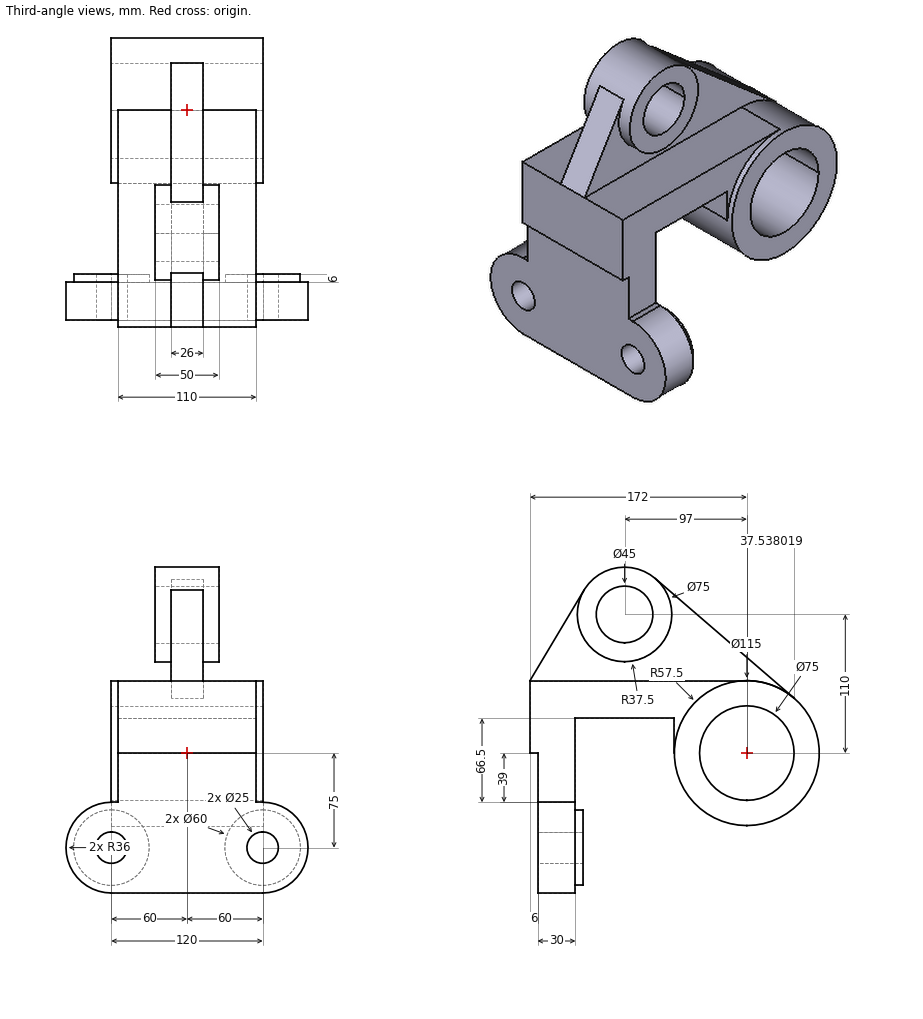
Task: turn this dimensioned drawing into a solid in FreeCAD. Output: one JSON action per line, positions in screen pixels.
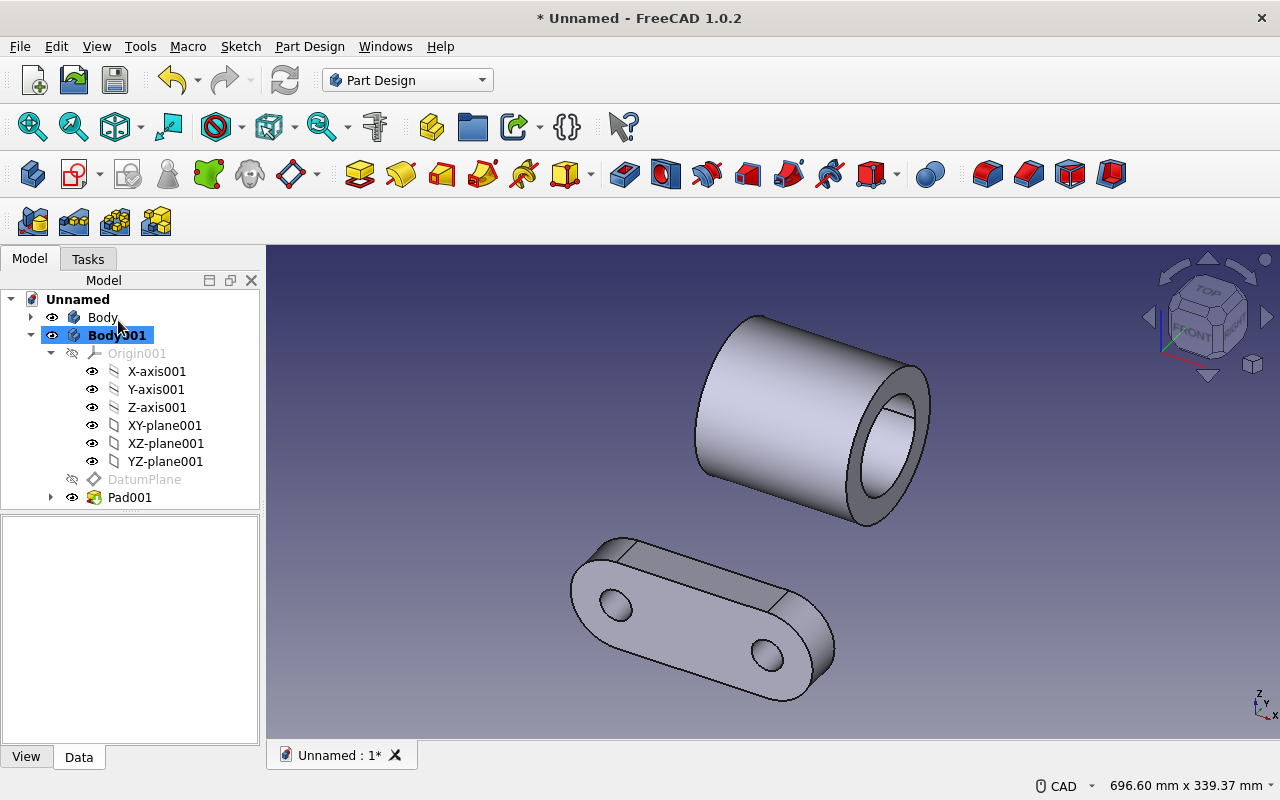
{"action": "key", "text": "4"}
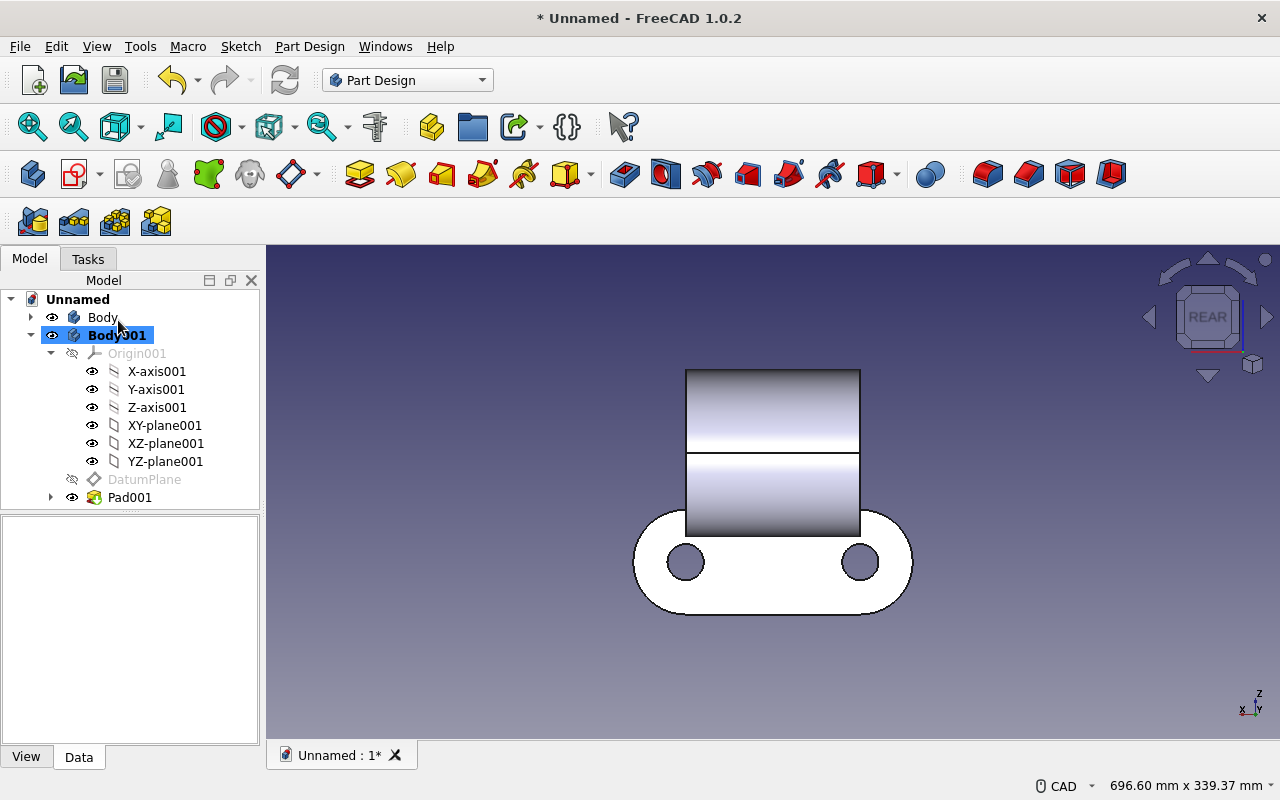
{"action": "left_click", "coordinate": [33, 128]}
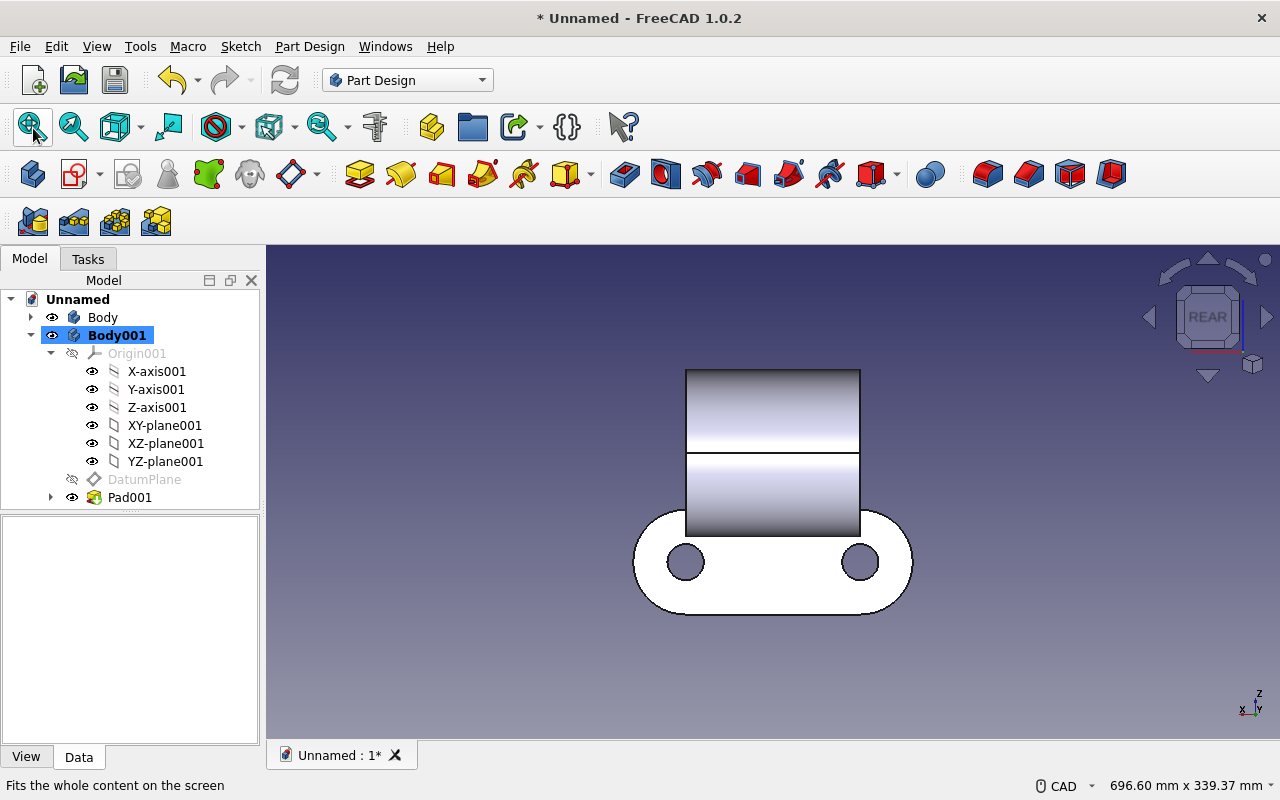
{"action": "left_click", "coordinate": [773, 561]}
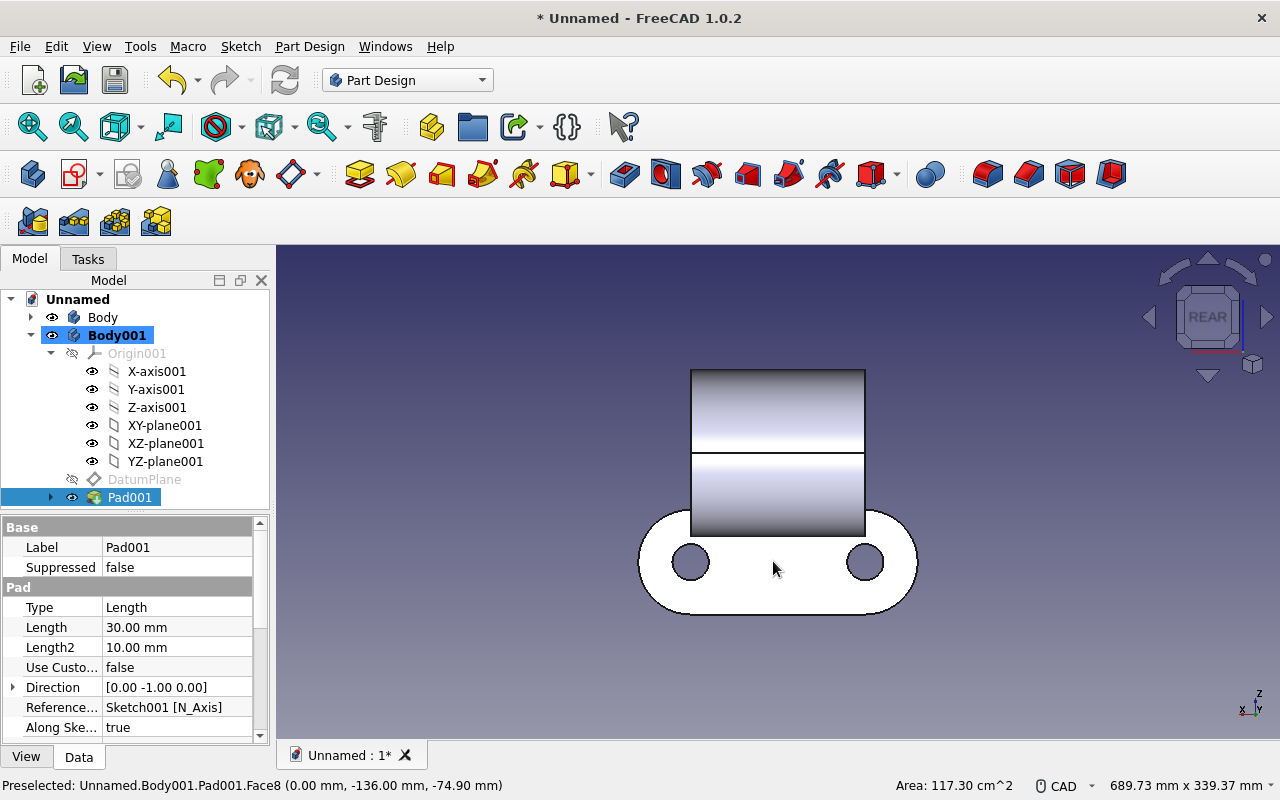
{"action": "left_click", "coordinate": [74, 174]}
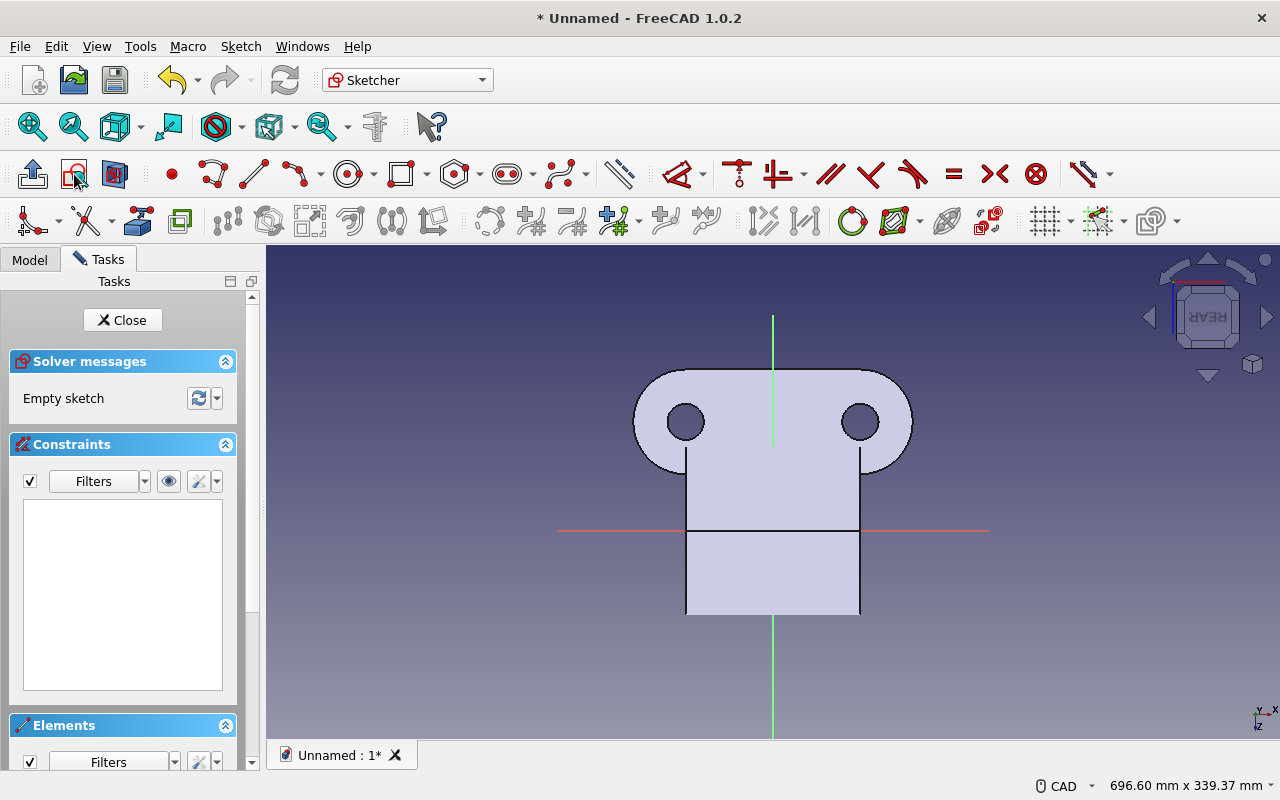
{"action": "scroll", "coordinate": [829, 424], "scroll_direction": "up", "scroll_amount": 4}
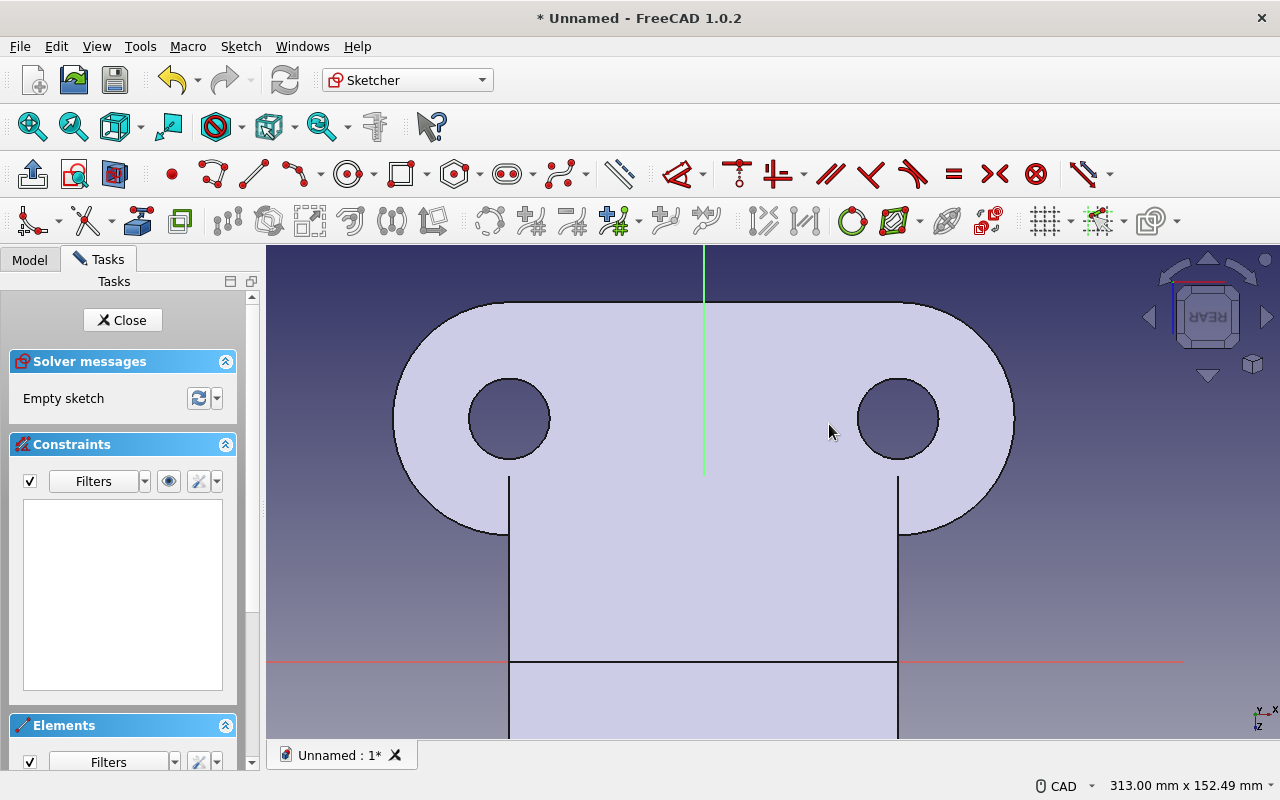
{"action": "left_click", "coordinate": [348, 174]}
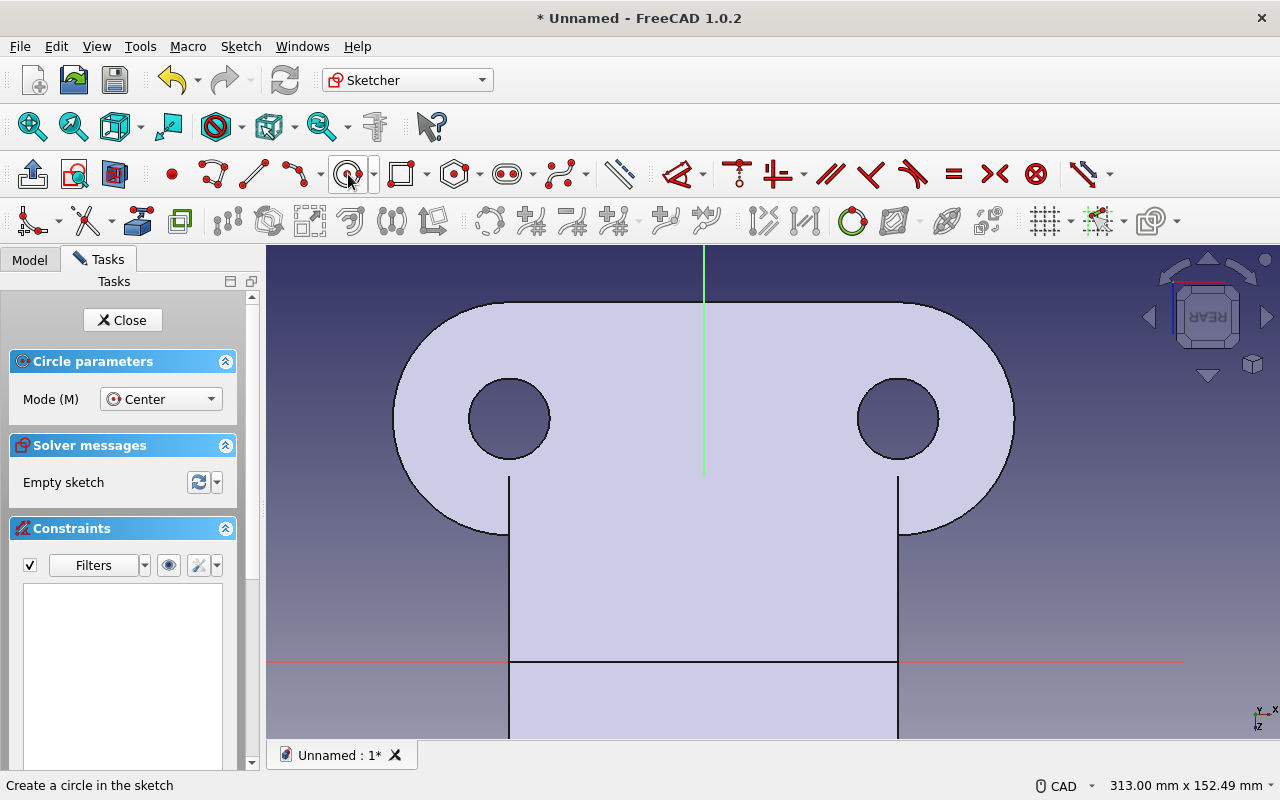
{"action": "left_click", "coordinate": [898, 419]}
{"action": "left_click", "coordinate": [967, 350]}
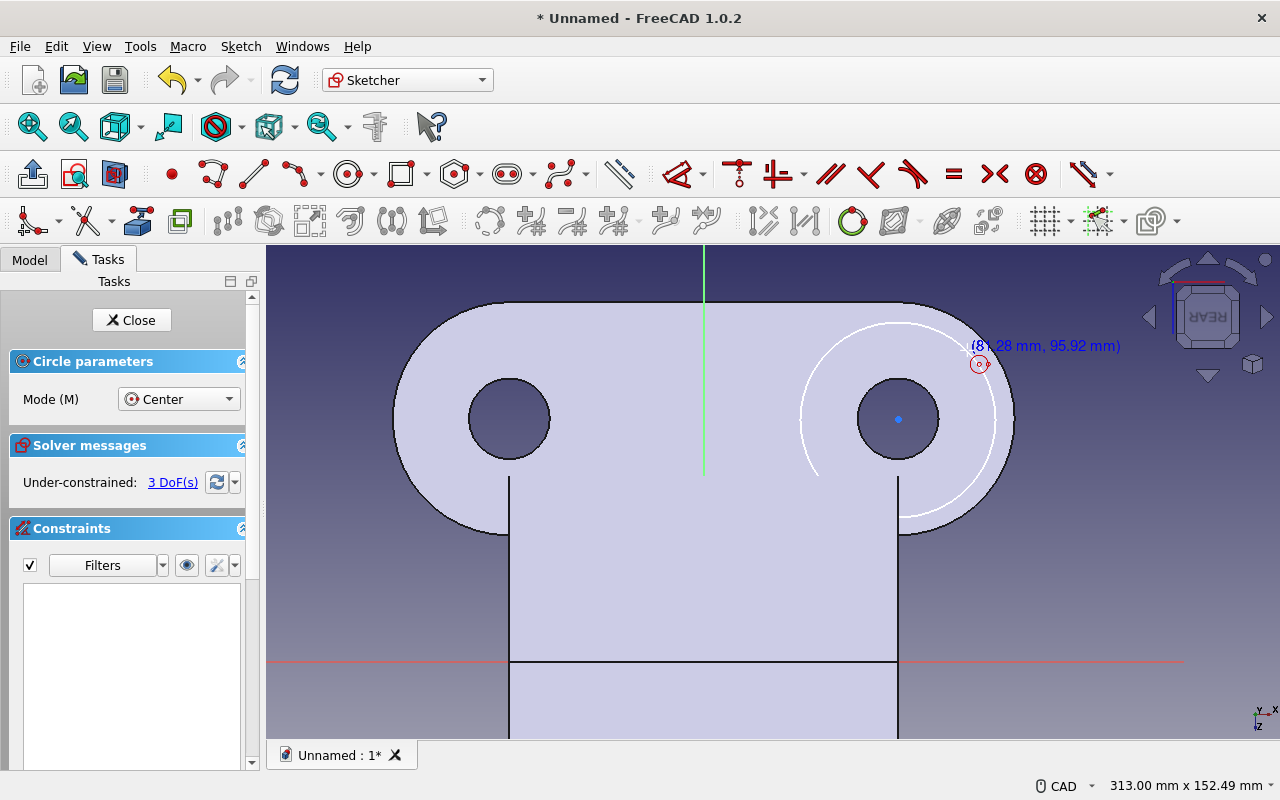
{"action": "left_click", "coordinate": [509, 419]}
{"action": "left_click", "coordinate": [578, 350]}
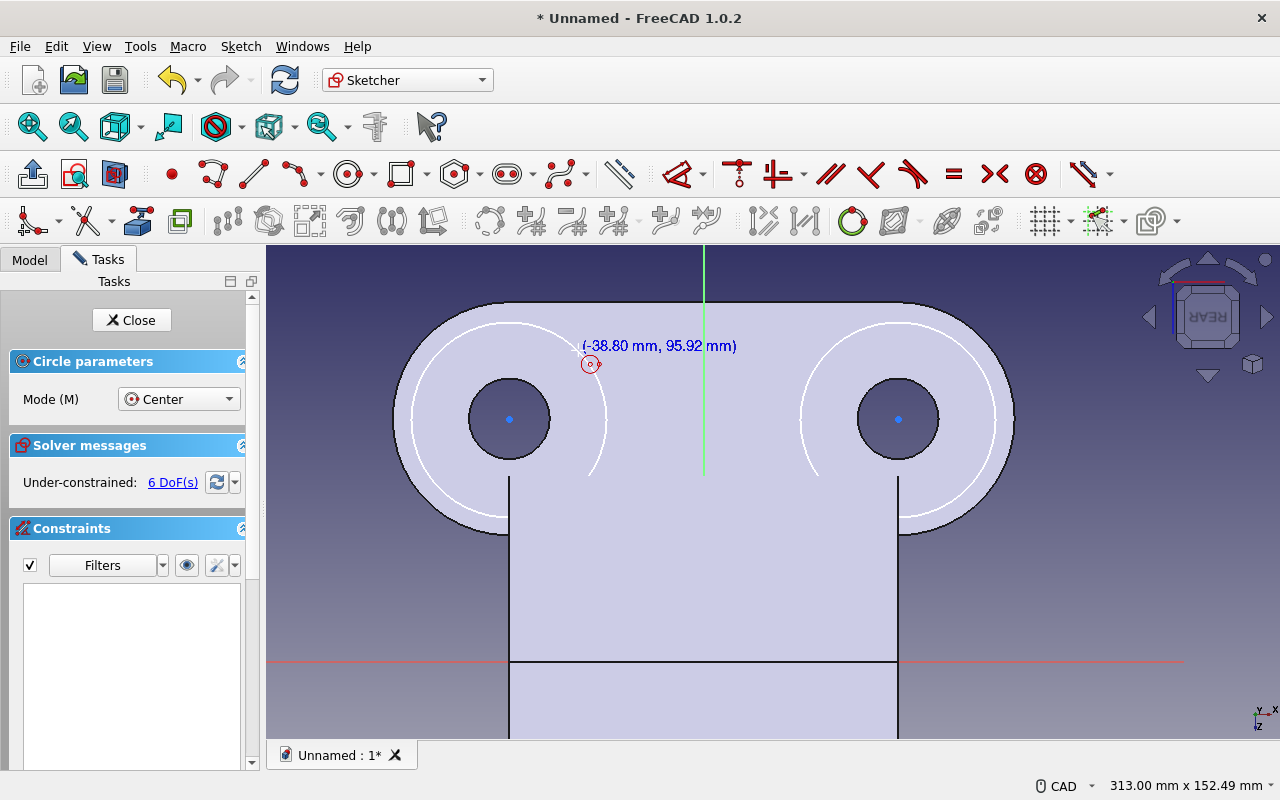
{"action": "left_click", "coordinate": [898, 420]}
{"action": "left_click", "coordinate": [927, 390]}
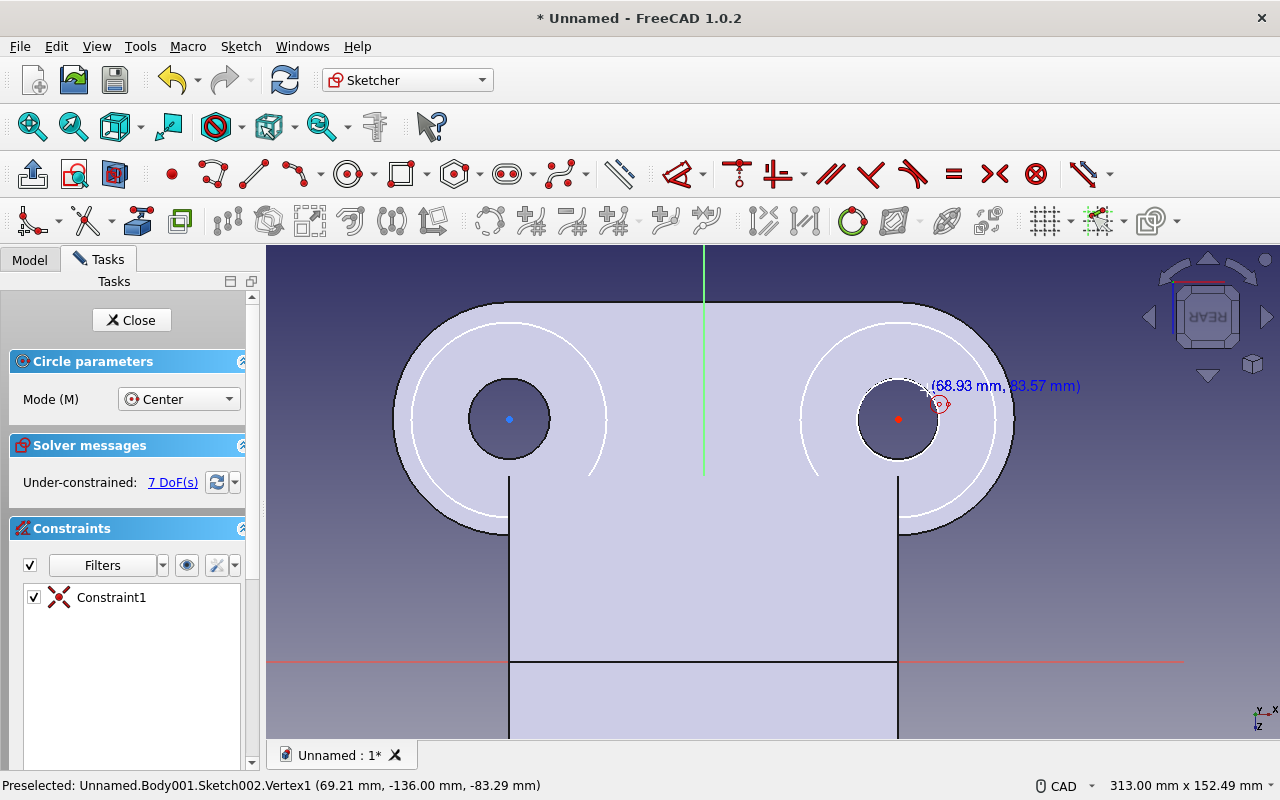
{"action": "left_click", "coordinate": [509, 420]}
{"action": "left_click", "coordinate": [538, 390]}
{"action": "key", "text": "Escape"}